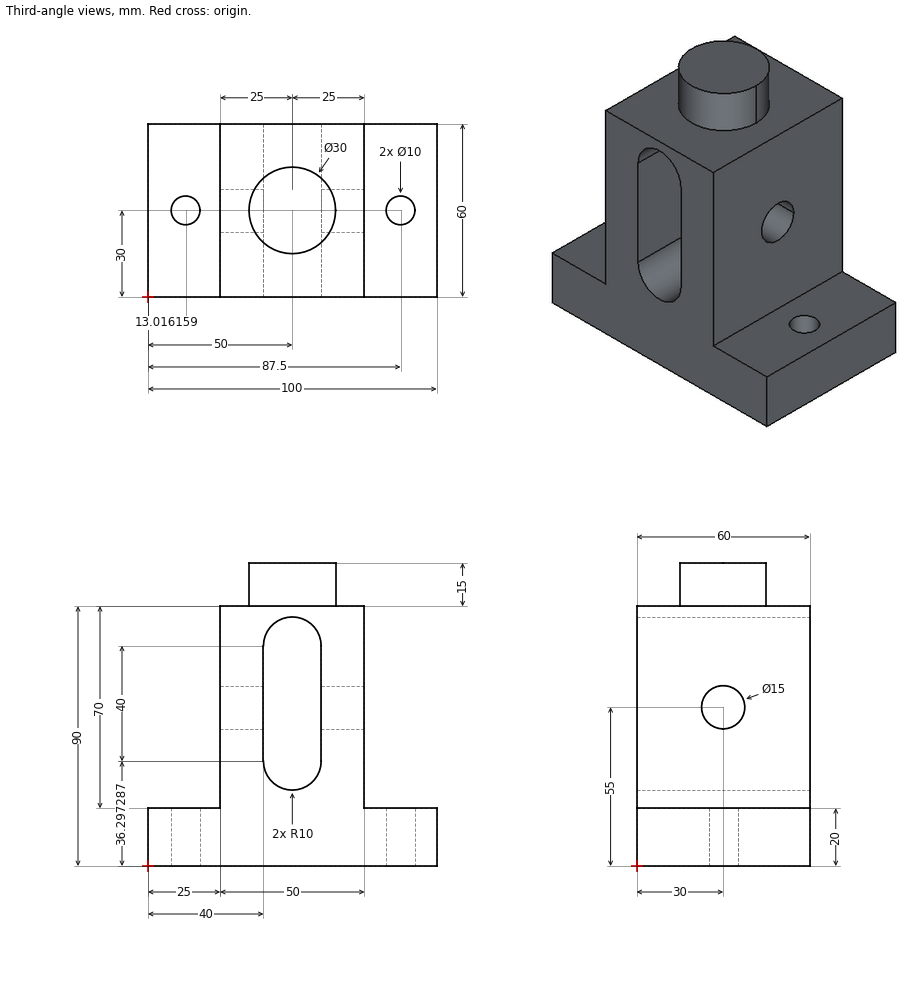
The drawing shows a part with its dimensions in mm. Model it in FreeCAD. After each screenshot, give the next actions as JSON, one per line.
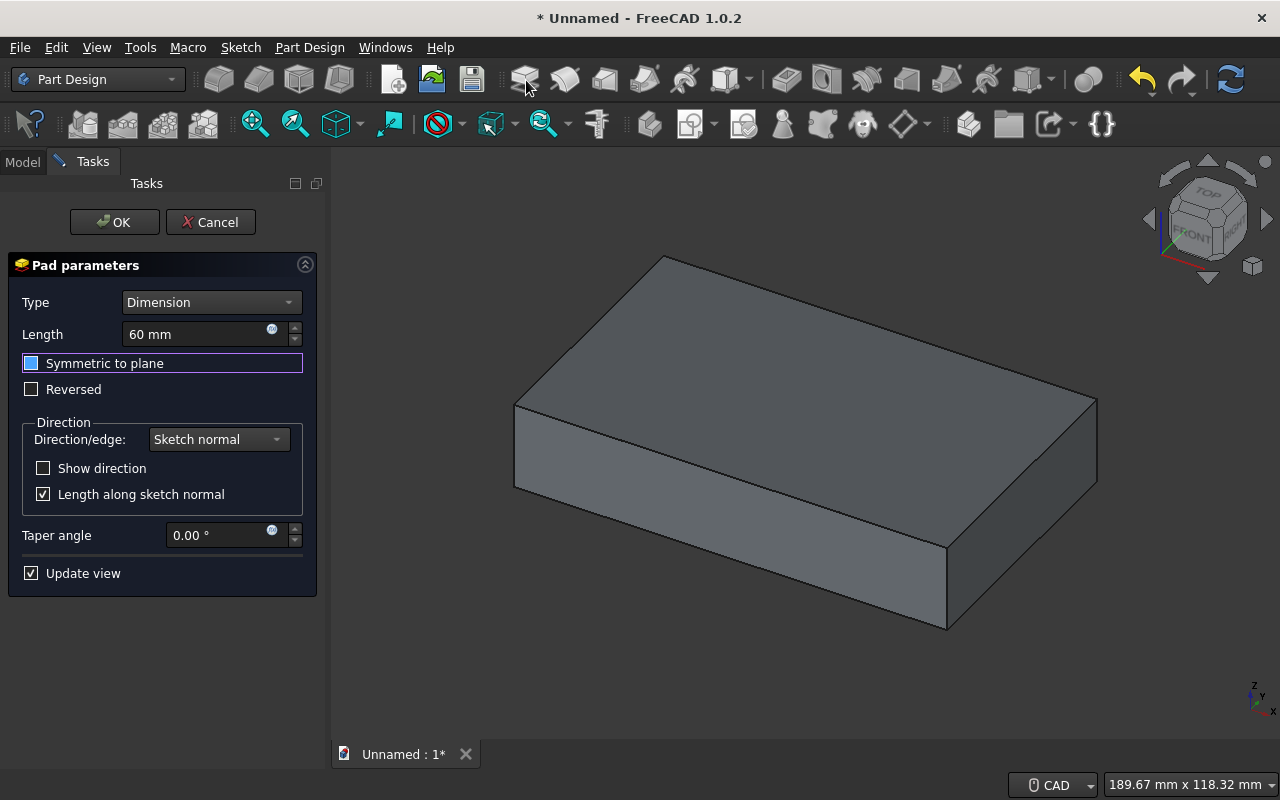
{"action": "left_click", "coordinate": [30, 389]}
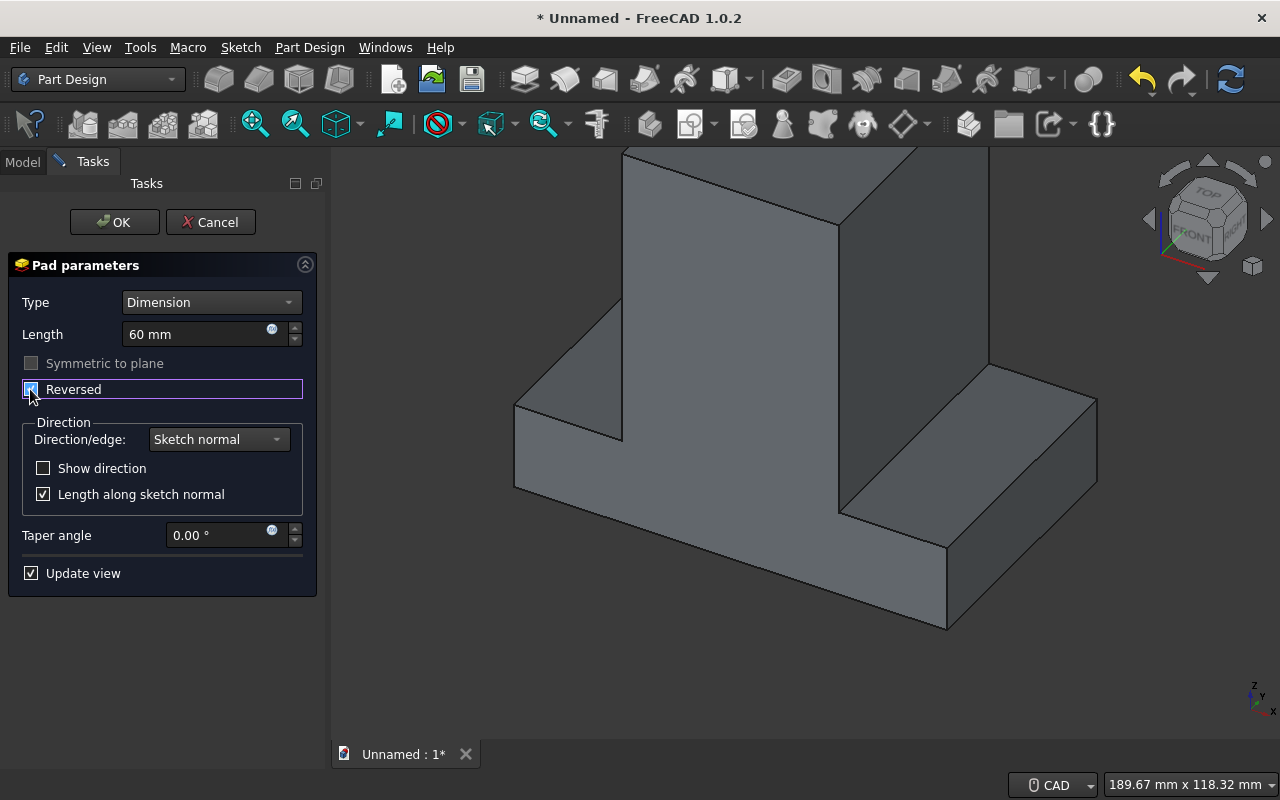
{"action": "left_click", "coordinate": [115, 222]}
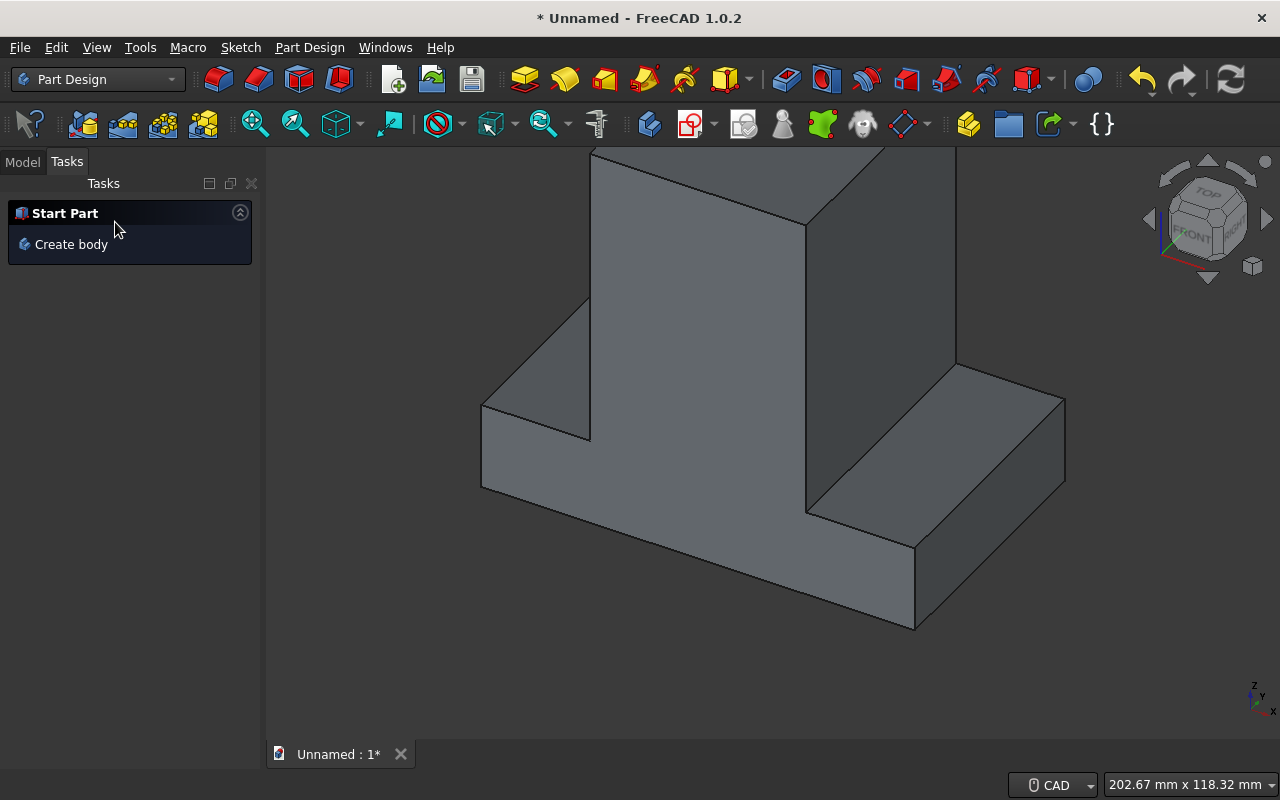
{"action": "key", "text": "v f"}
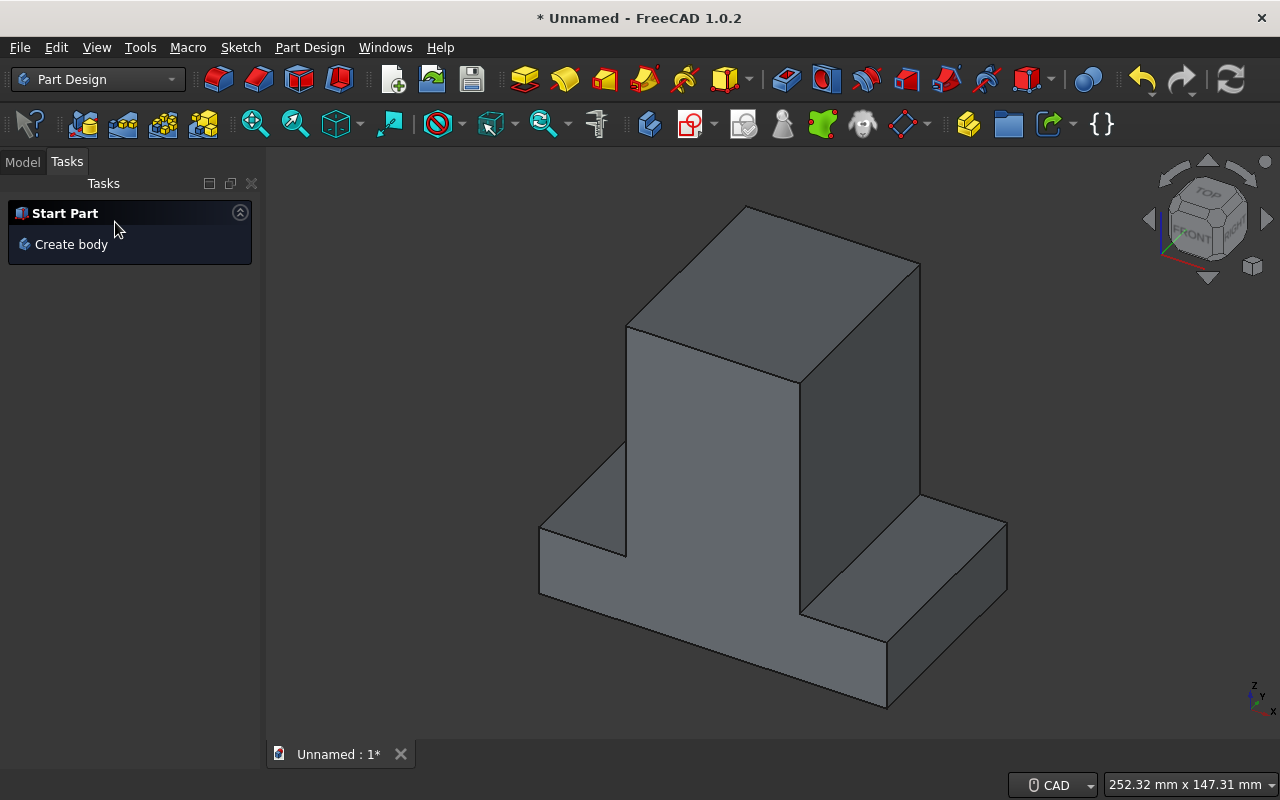
{"action": "left_click", "coordinate": [713, 460]}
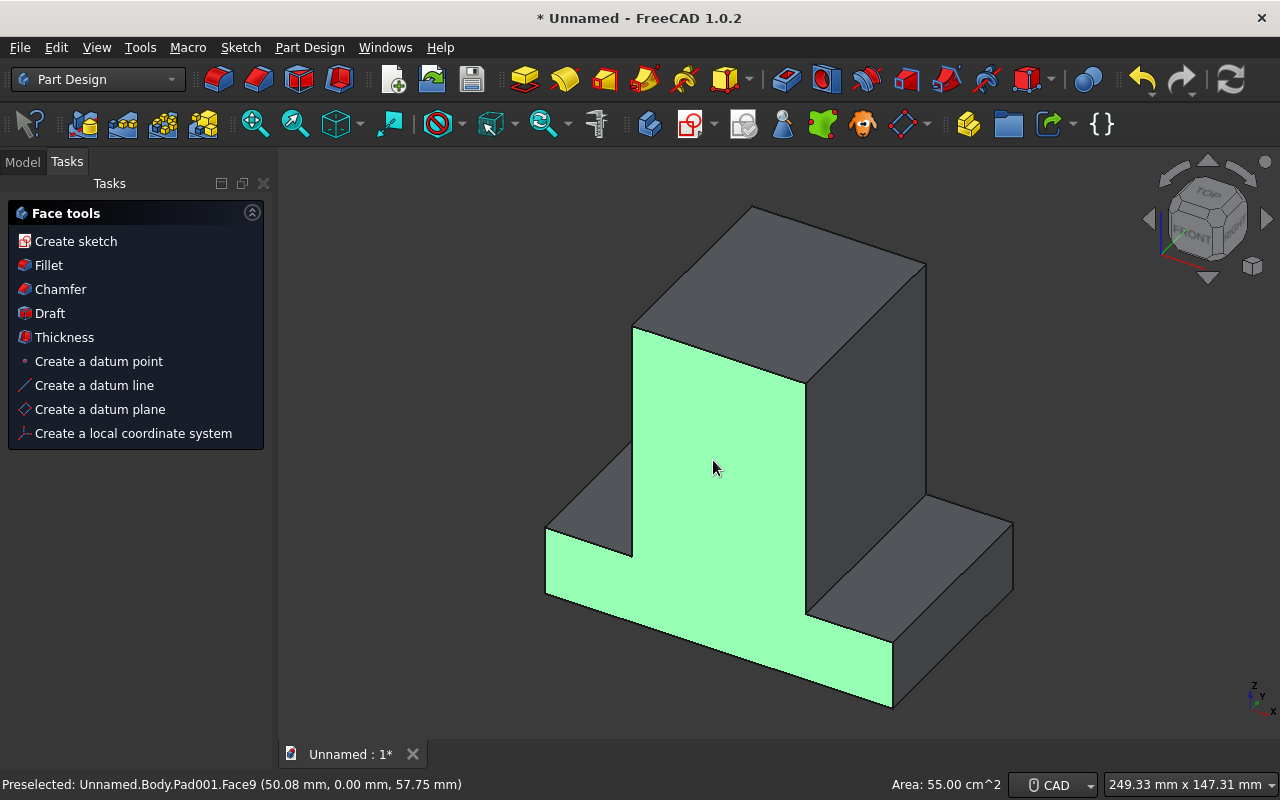
{"action": "left_click", "coordinate": [690, 124]}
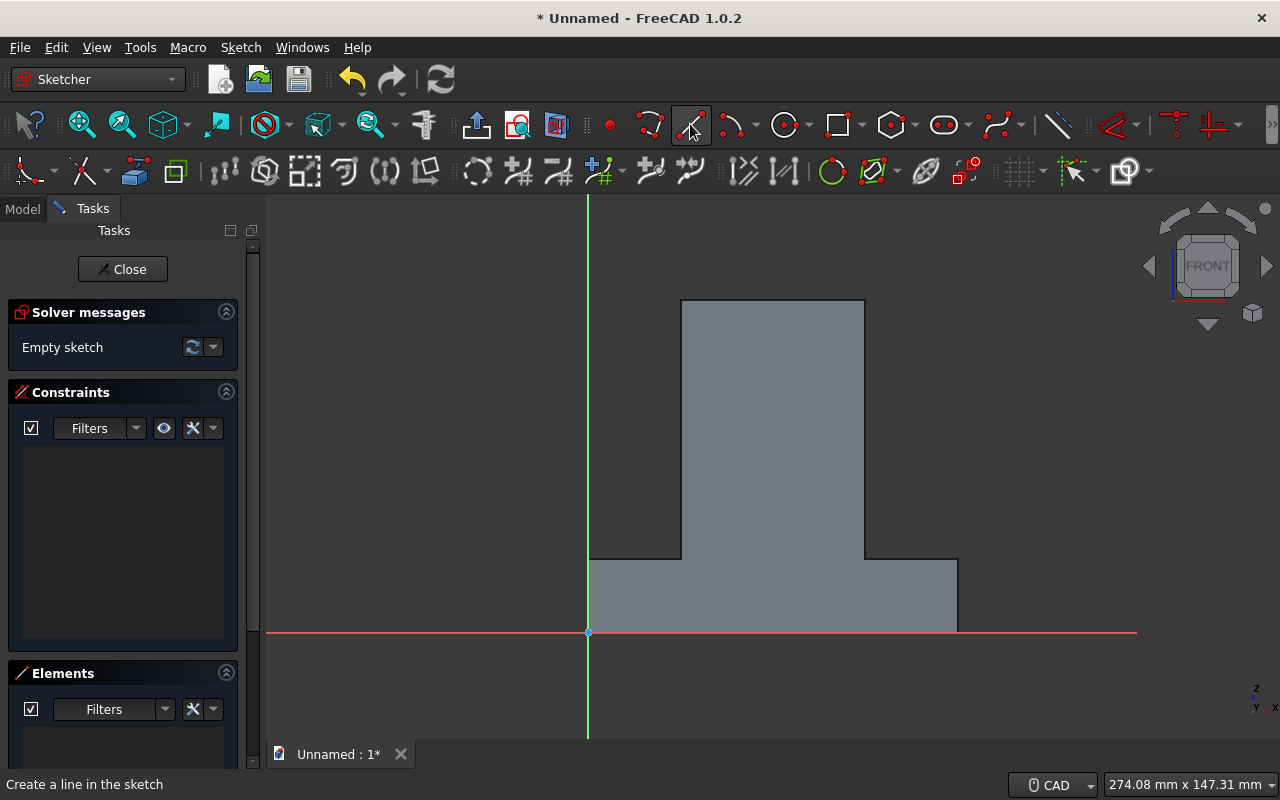
{"action": "key", "text": "g s"}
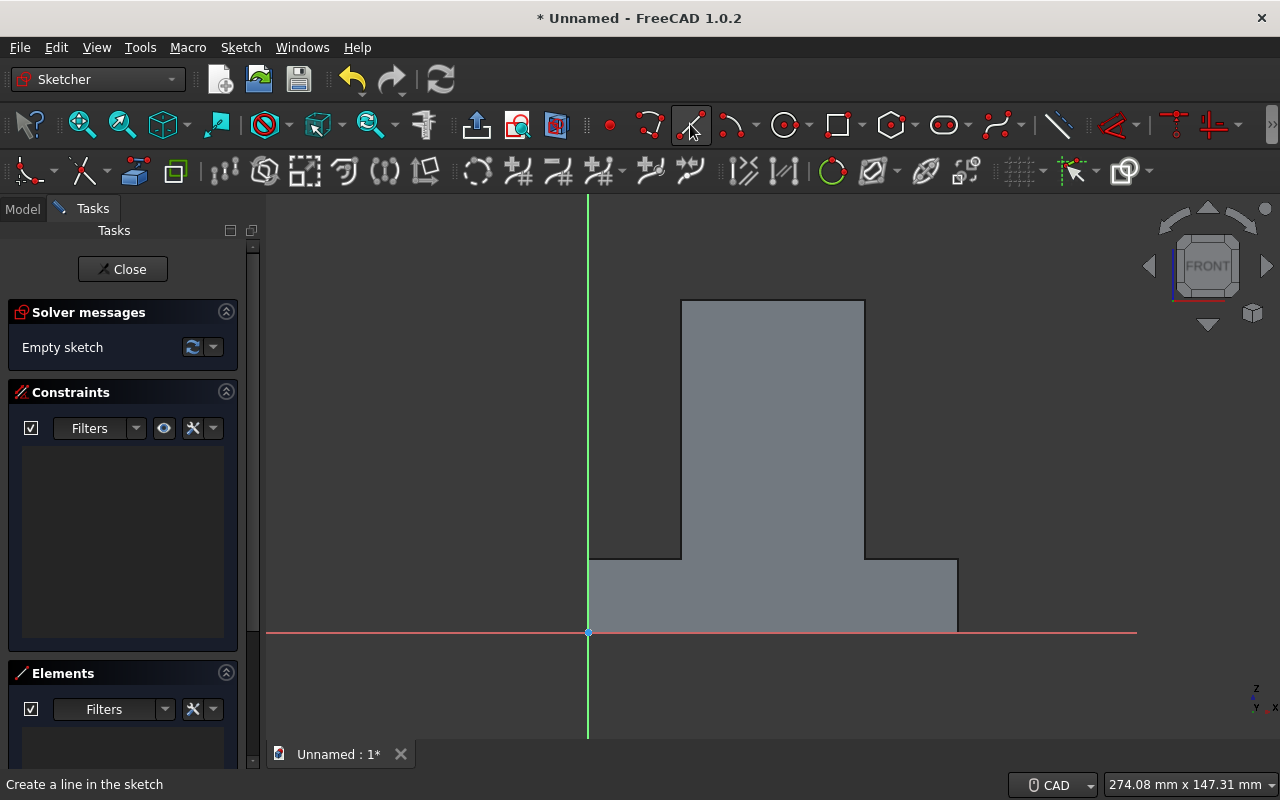
{"action": "left_click", "coordinate": [773, 499]}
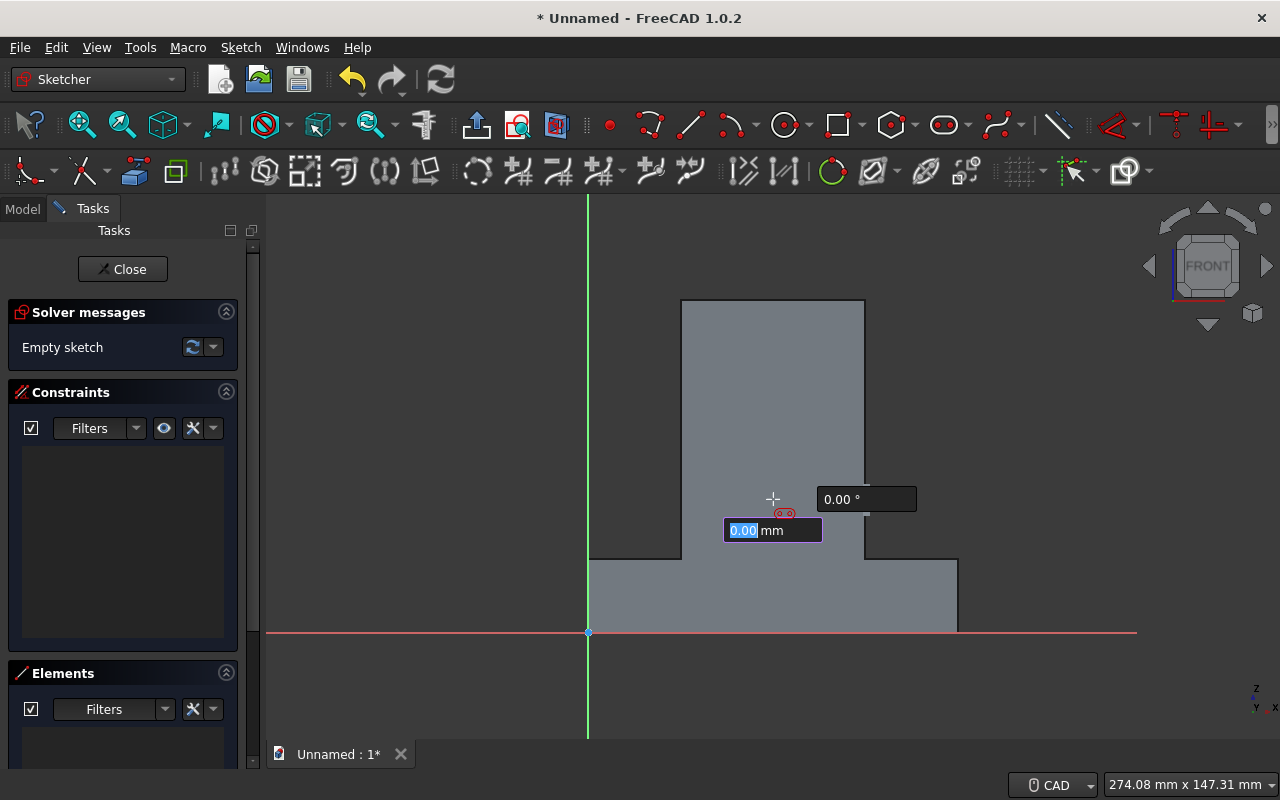
{"action": "left_click", "coordinate": [773, 351]}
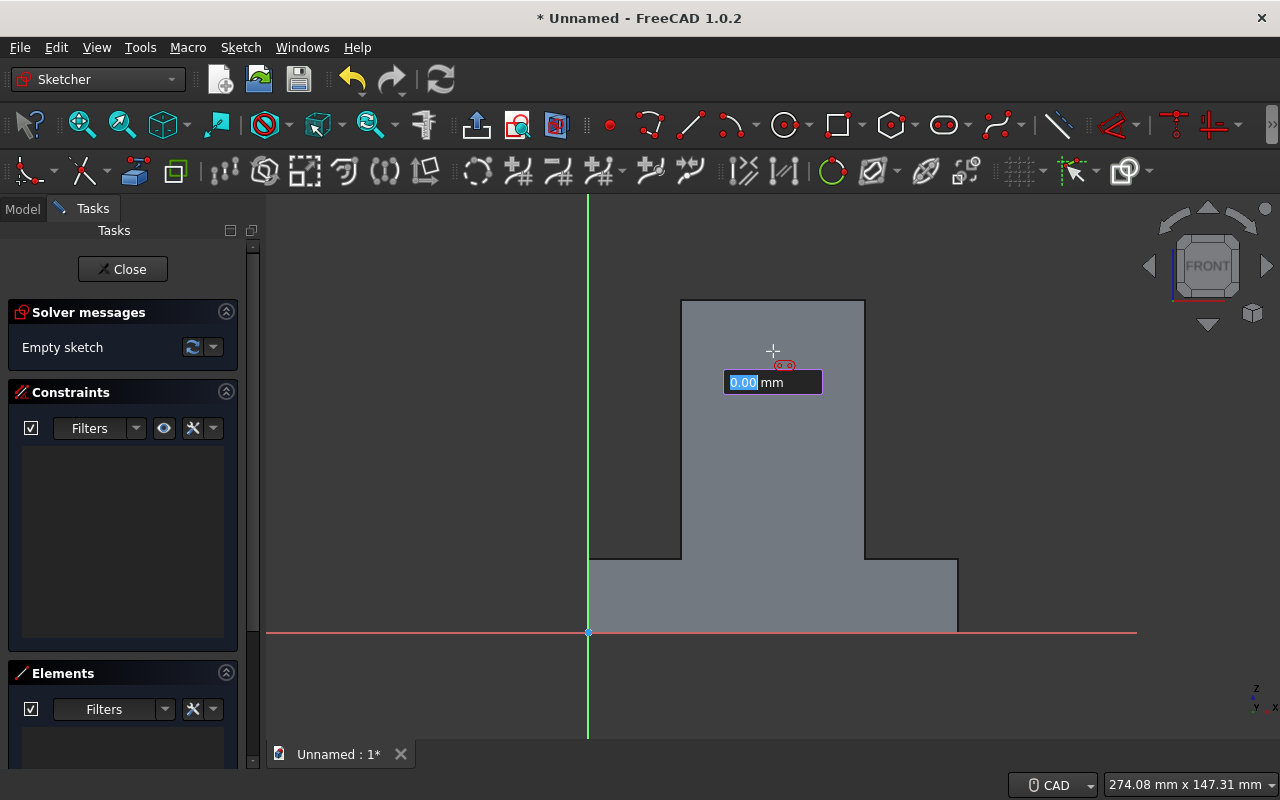
{"action": "left_click", "coordinate": [736, 425]}
{"action": "key", "text": "Escape"}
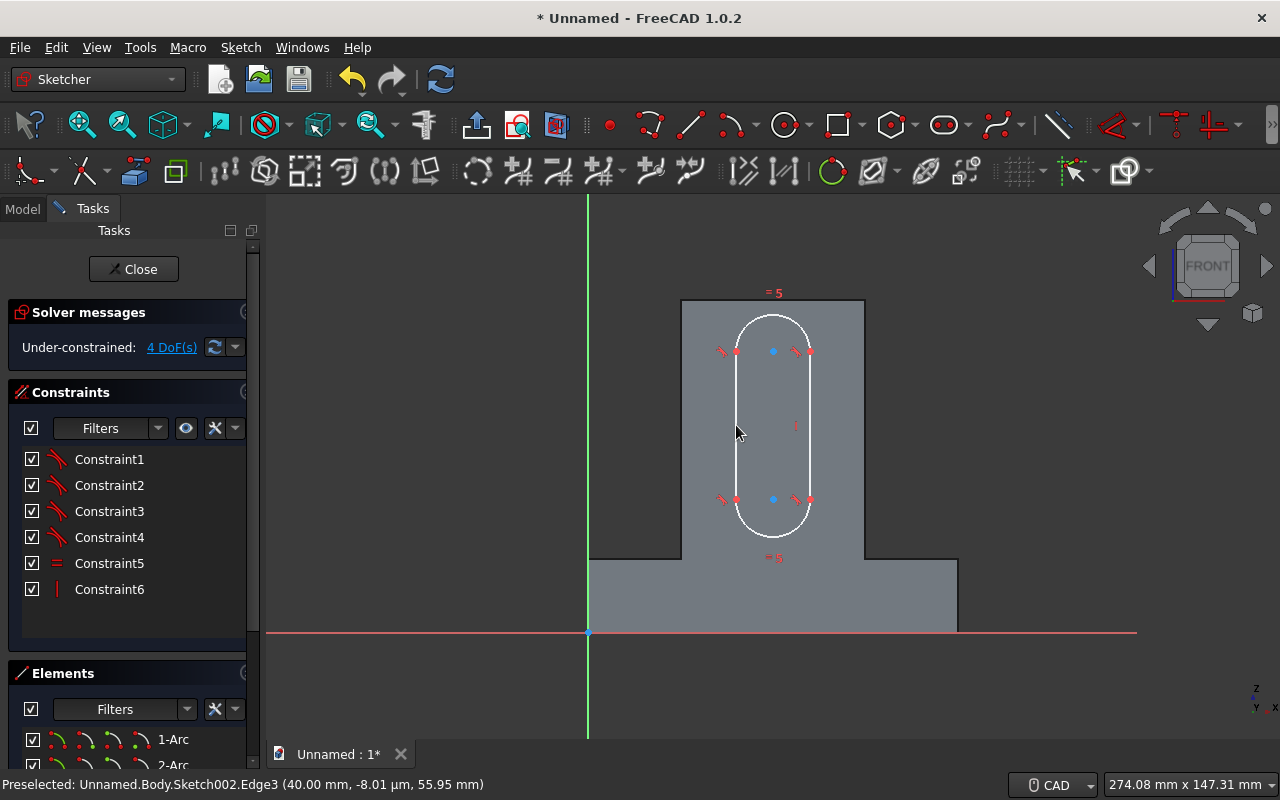
{"action": "left_click", "coordinate": [751, 530]}